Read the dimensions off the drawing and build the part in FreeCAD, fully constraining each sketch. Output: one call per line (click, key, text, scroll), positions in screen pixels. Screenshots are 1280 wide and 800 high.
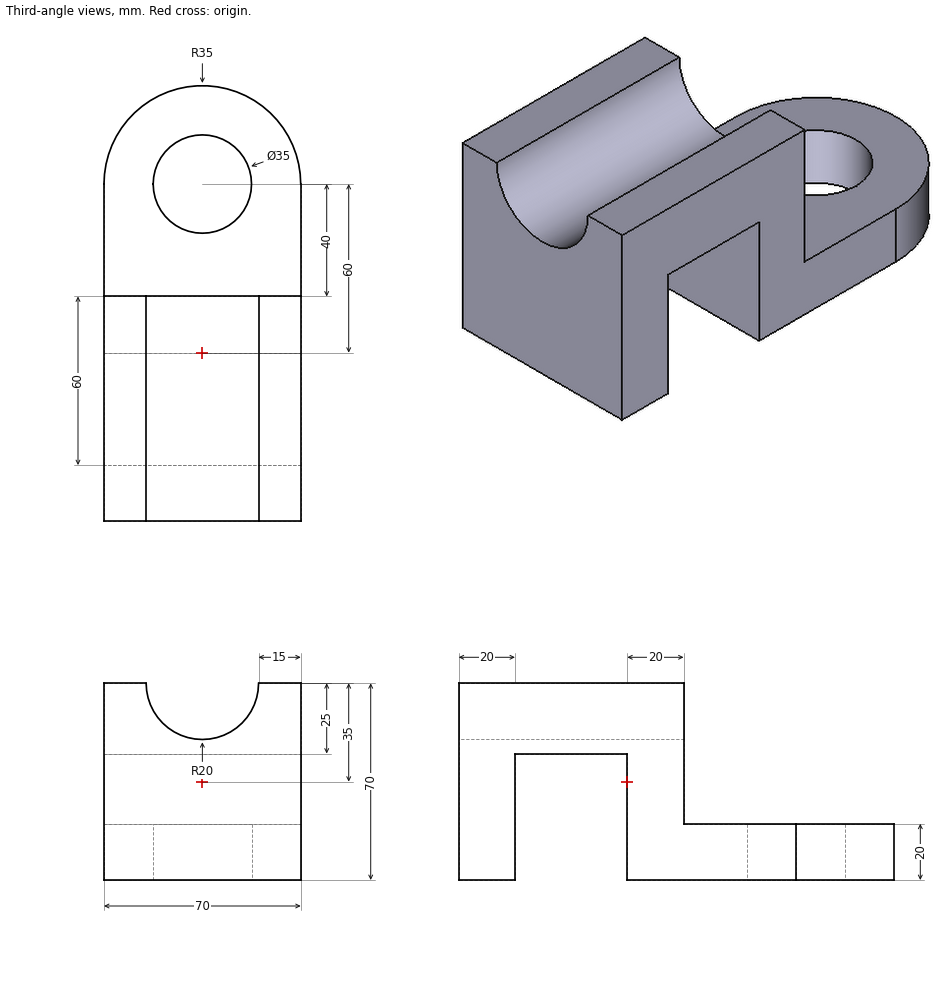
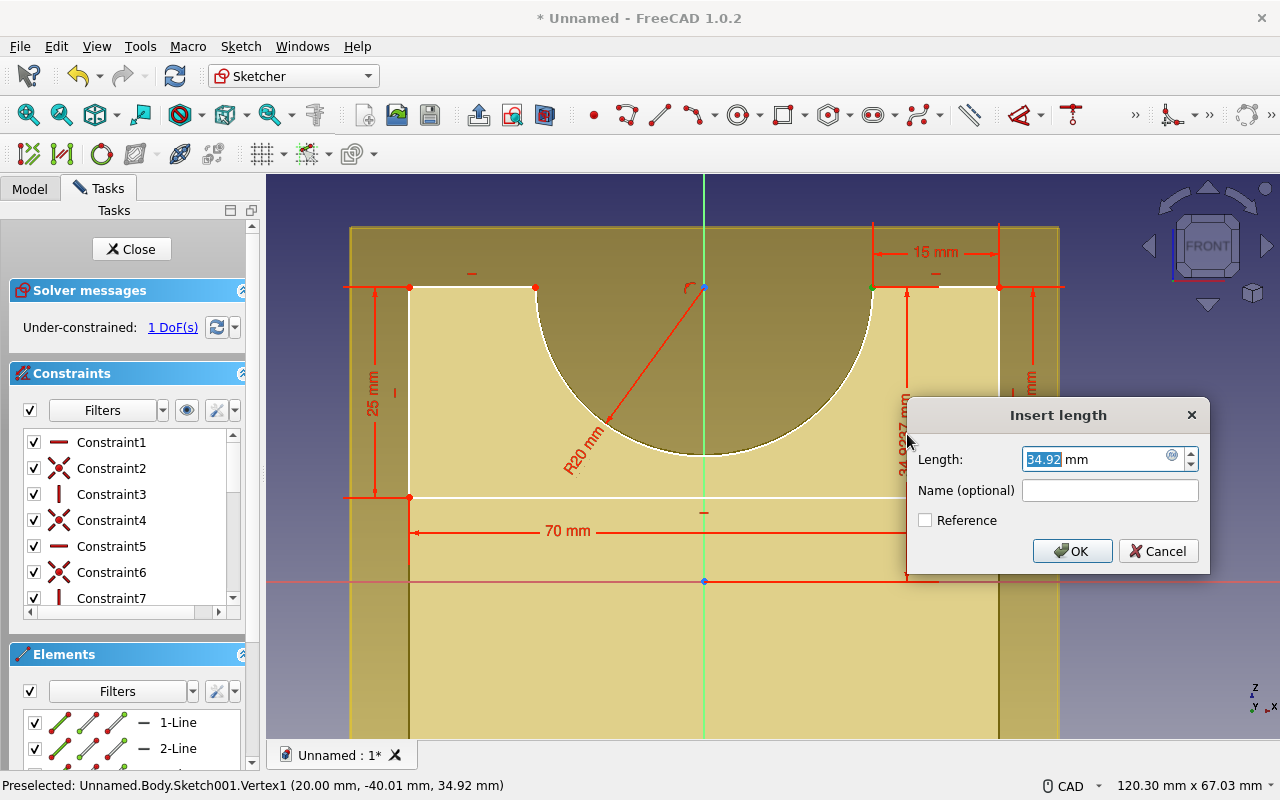
text(35)
key(Return)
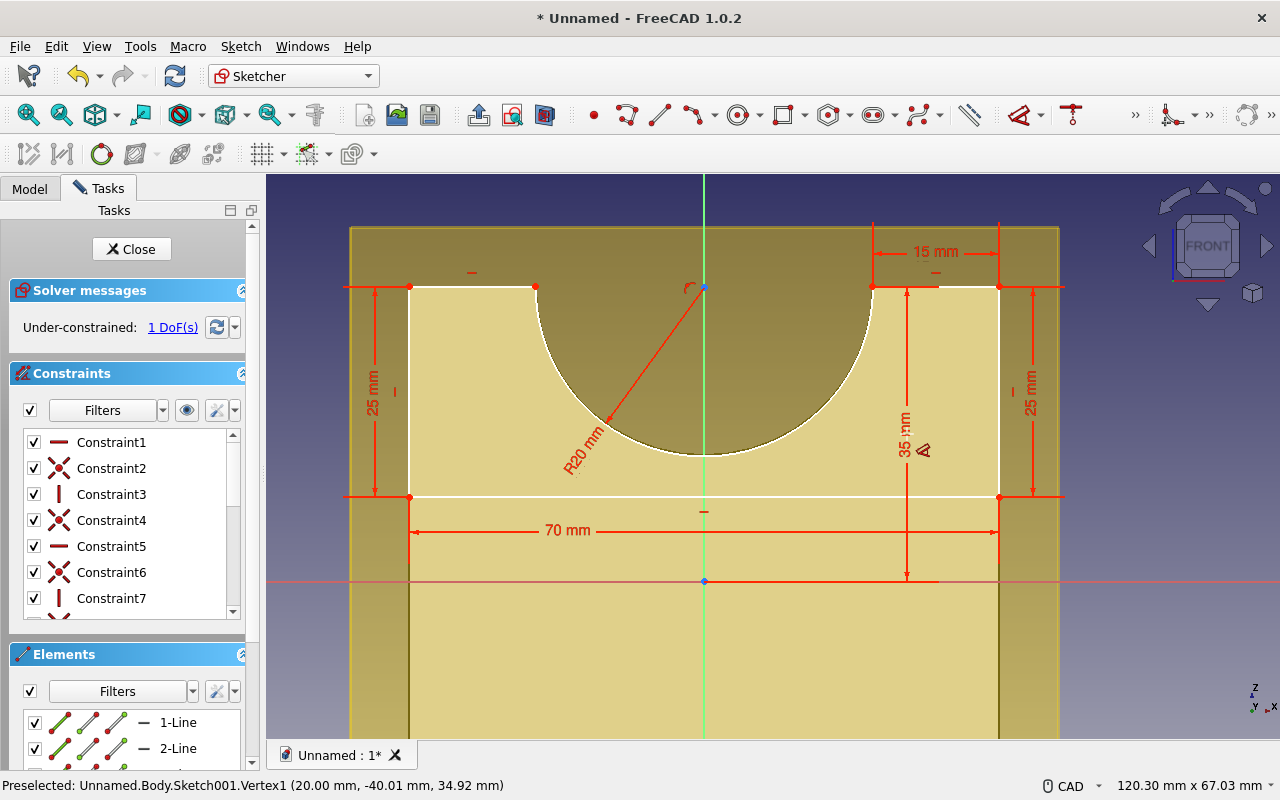
click(704, 288)
click(738, 435)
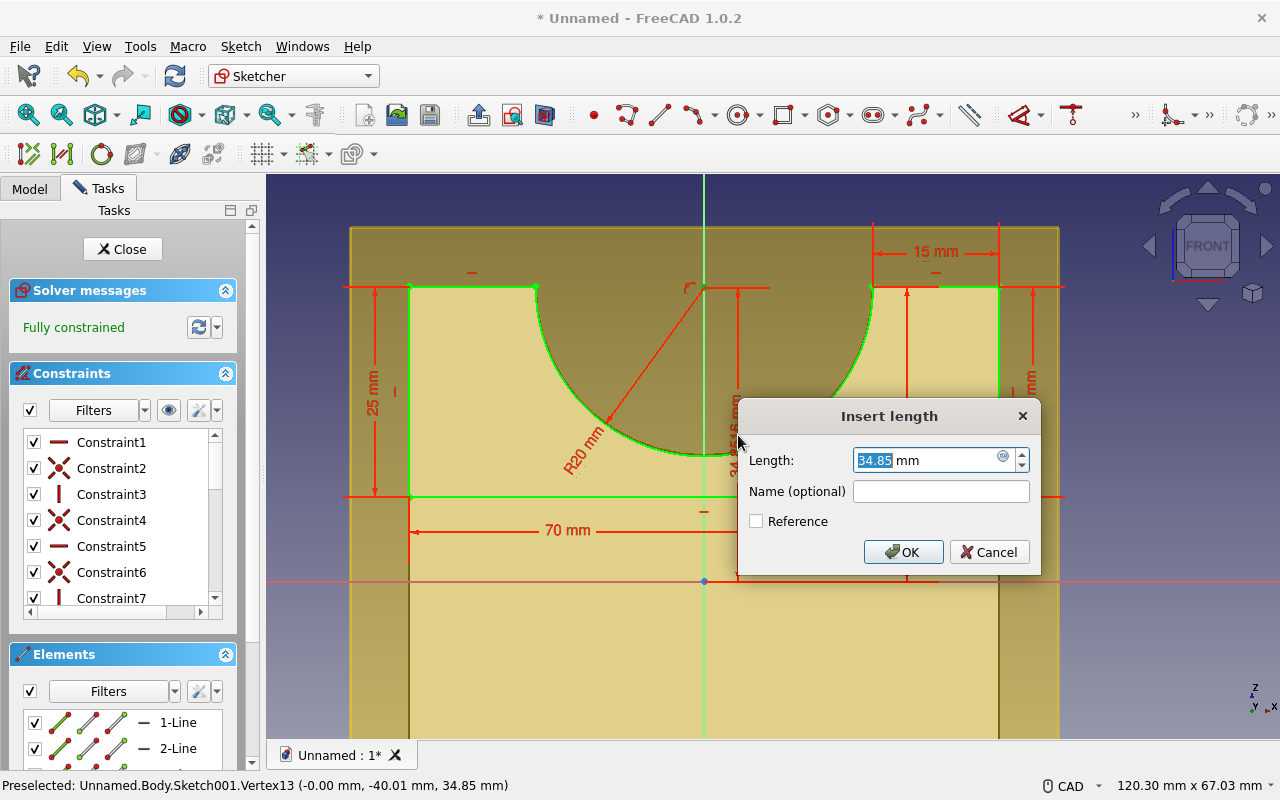
text(35)
key(Return)
key(Escape)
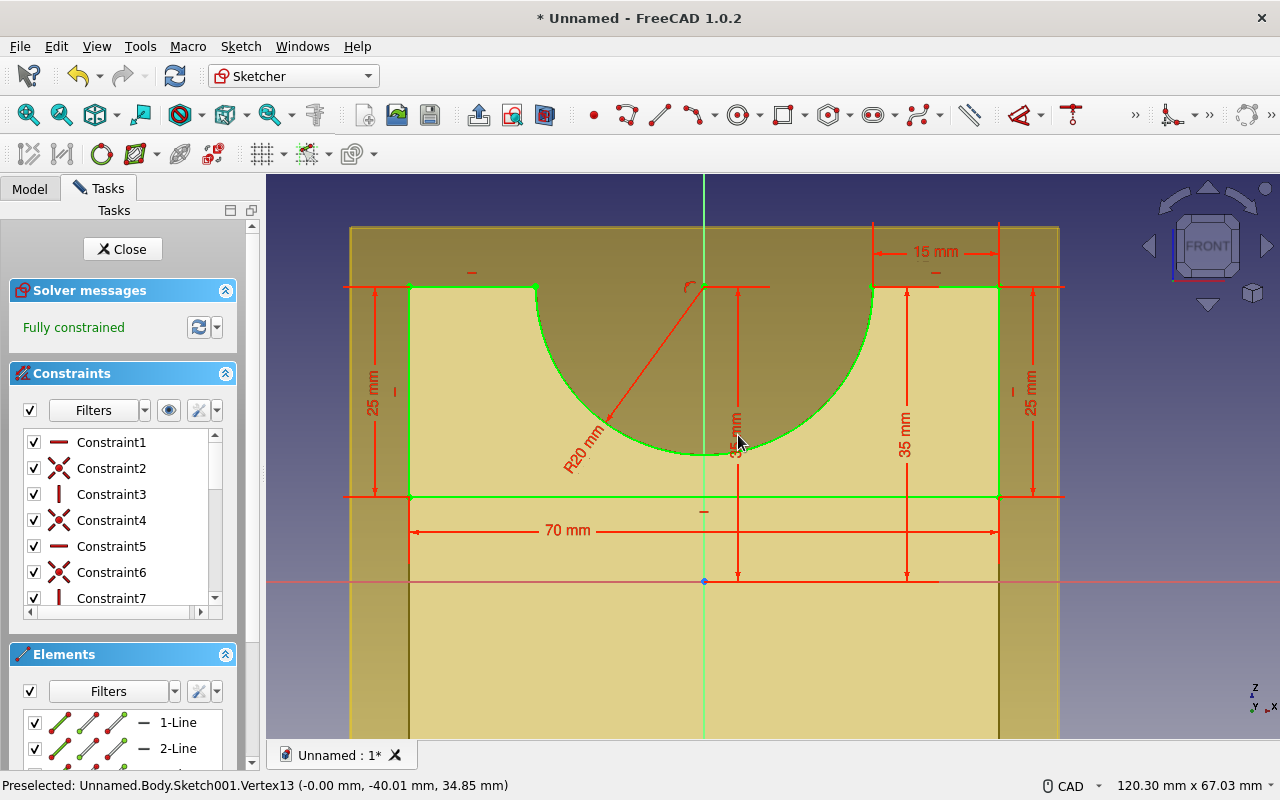
click(123, 249)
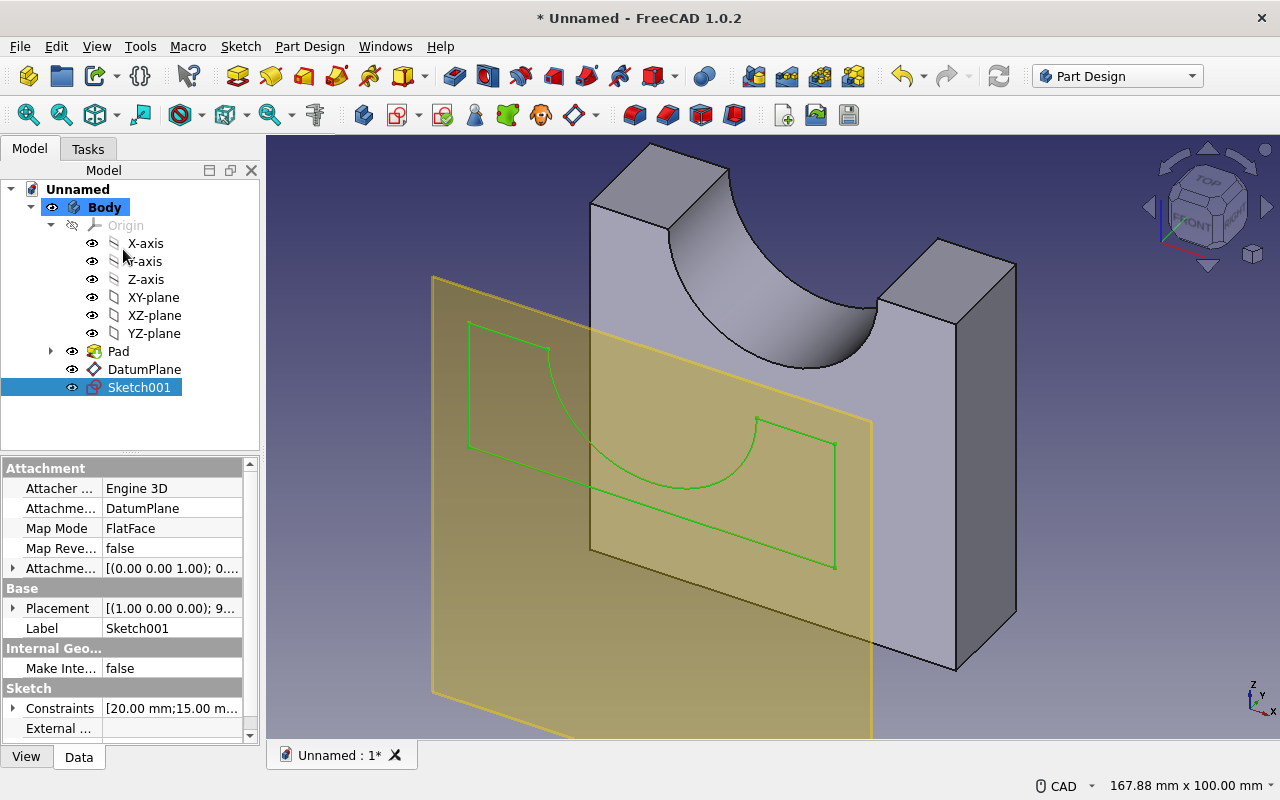
click(238, 76)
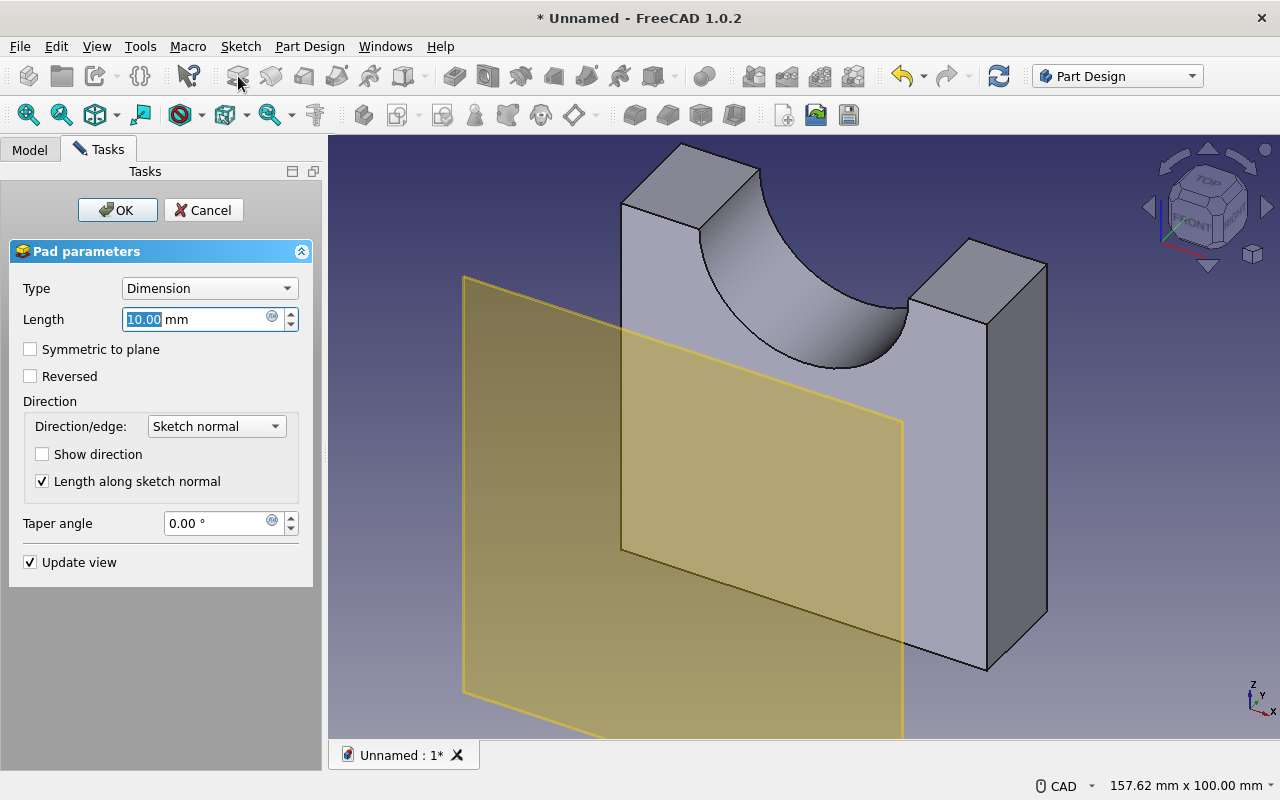
text(60)
key(Tab)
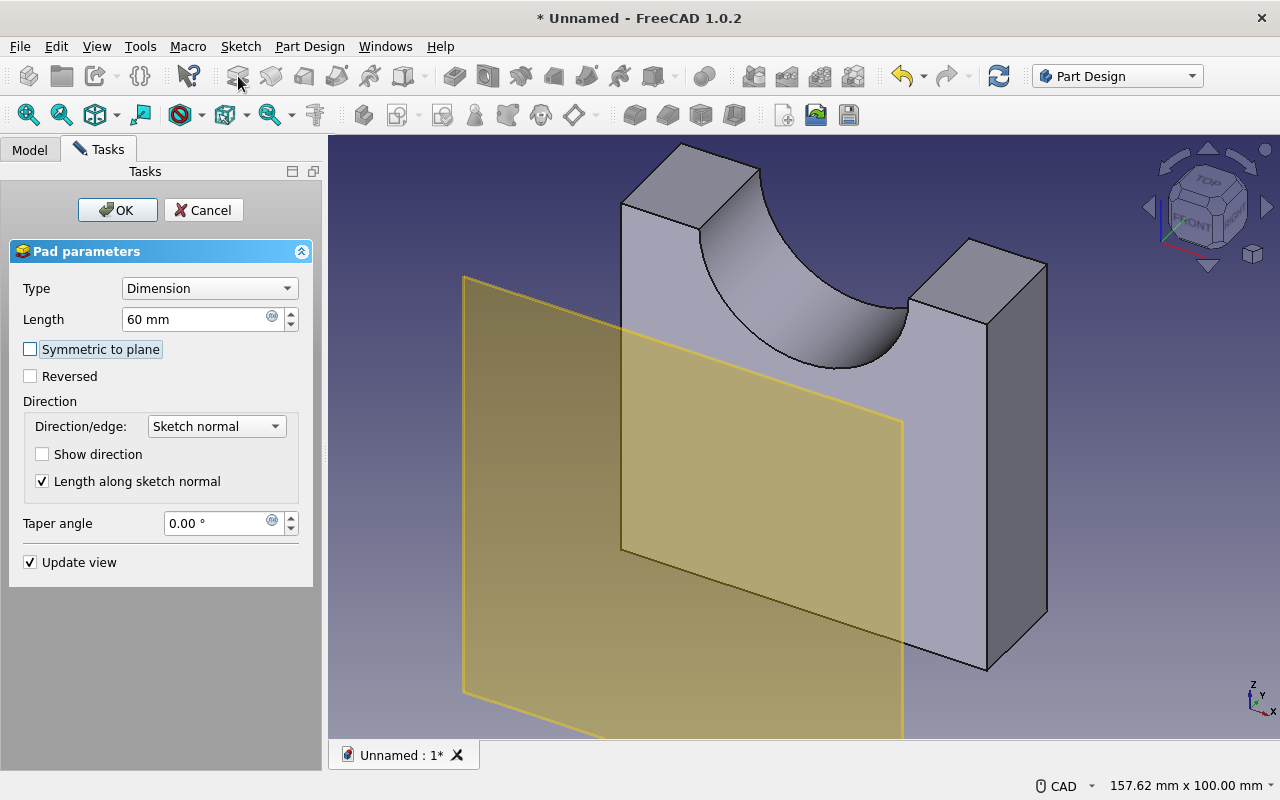
click(31, 376)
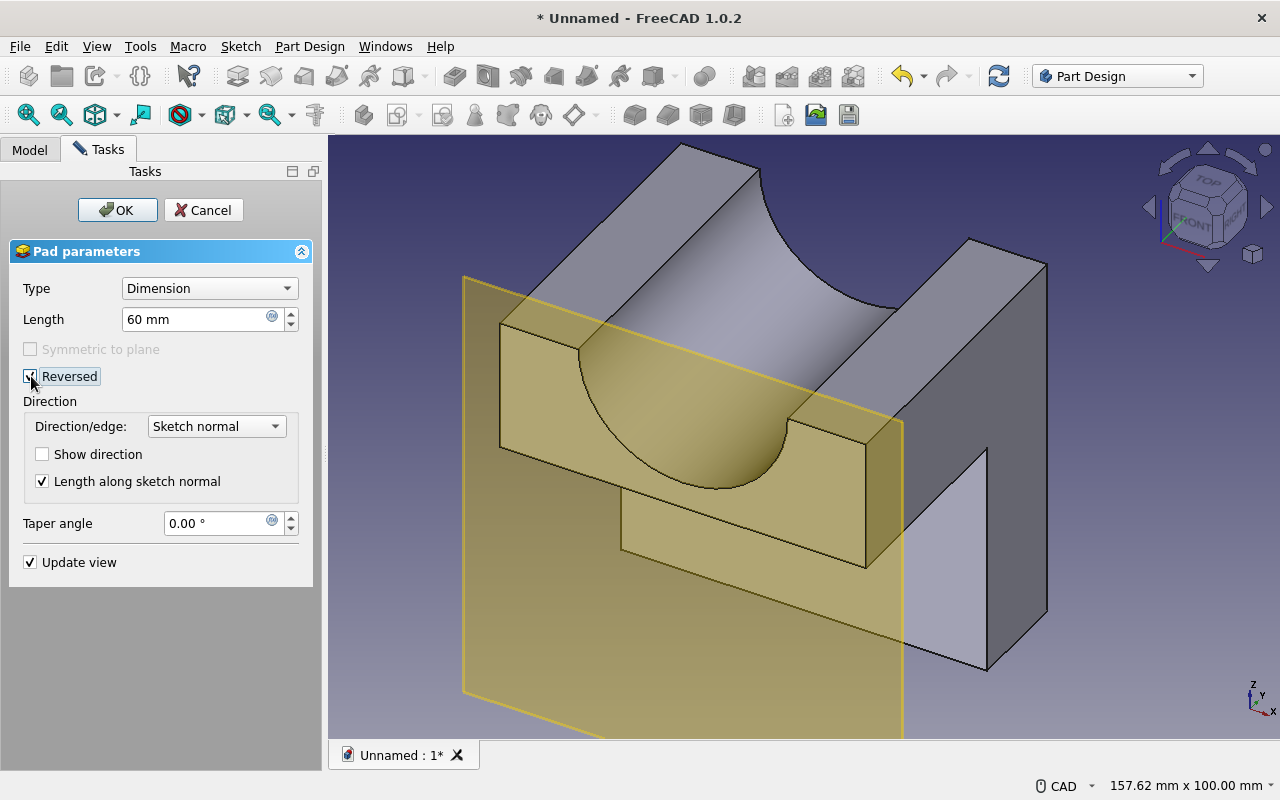
click(118, 210)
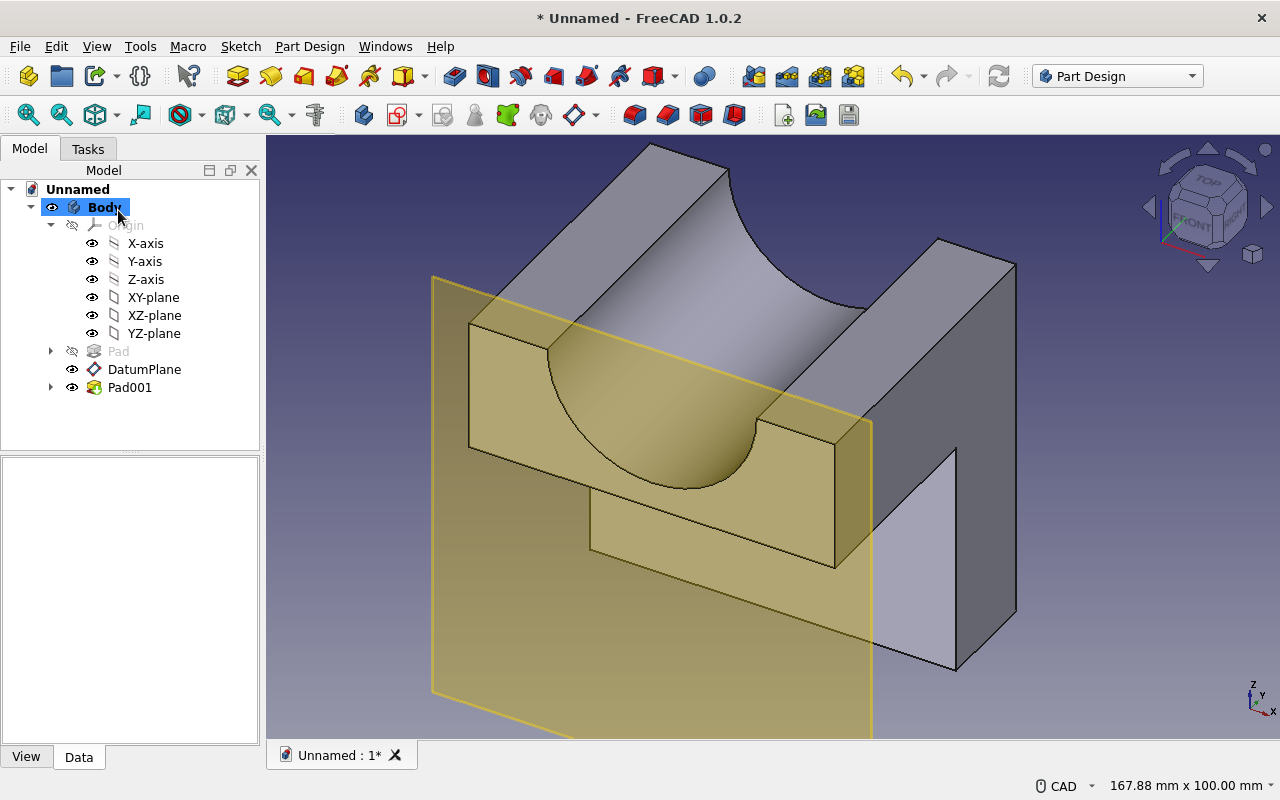
click(117, 369)
key(space)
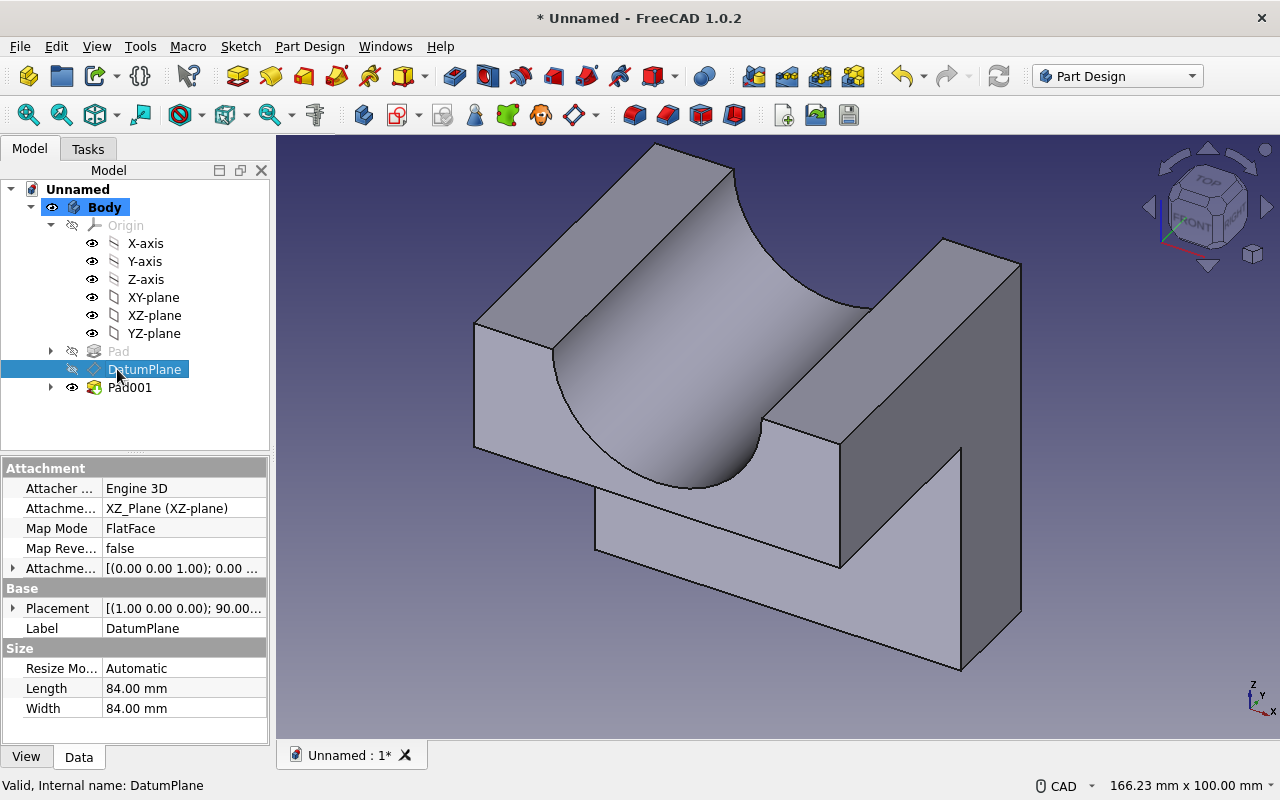
click(29, 116)